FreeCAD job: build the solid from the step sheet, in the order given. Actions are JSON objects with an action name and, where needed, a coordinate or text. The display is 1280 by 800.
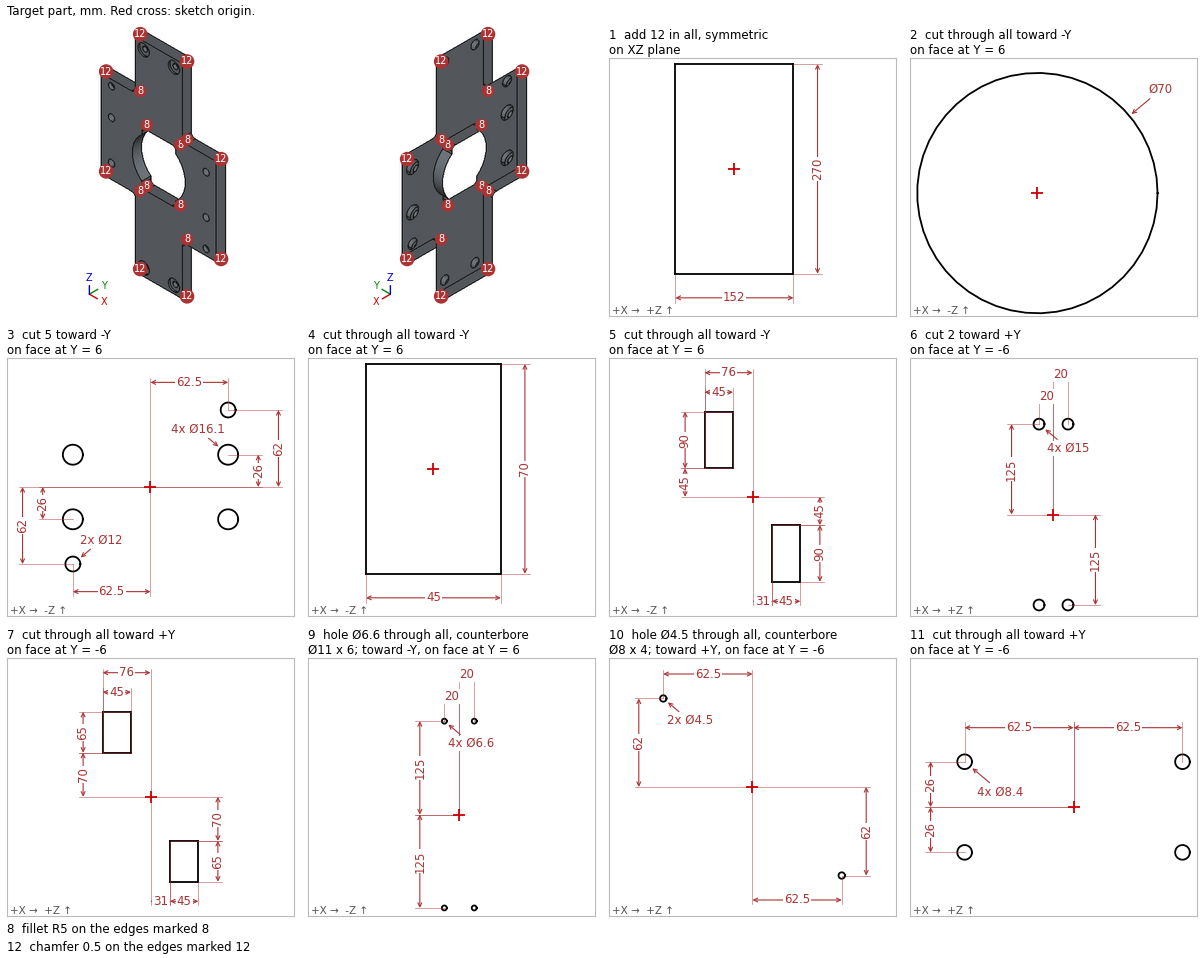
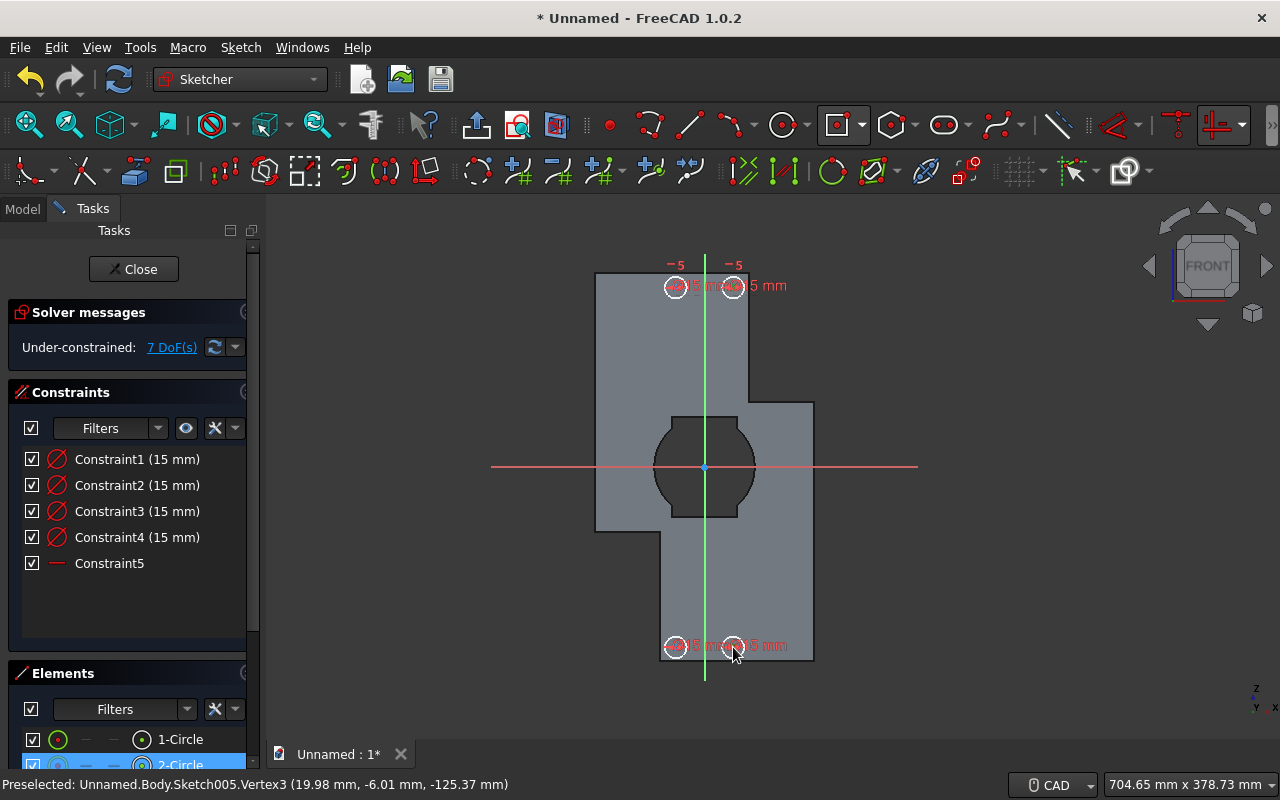
{"action": "key", "text": "v"}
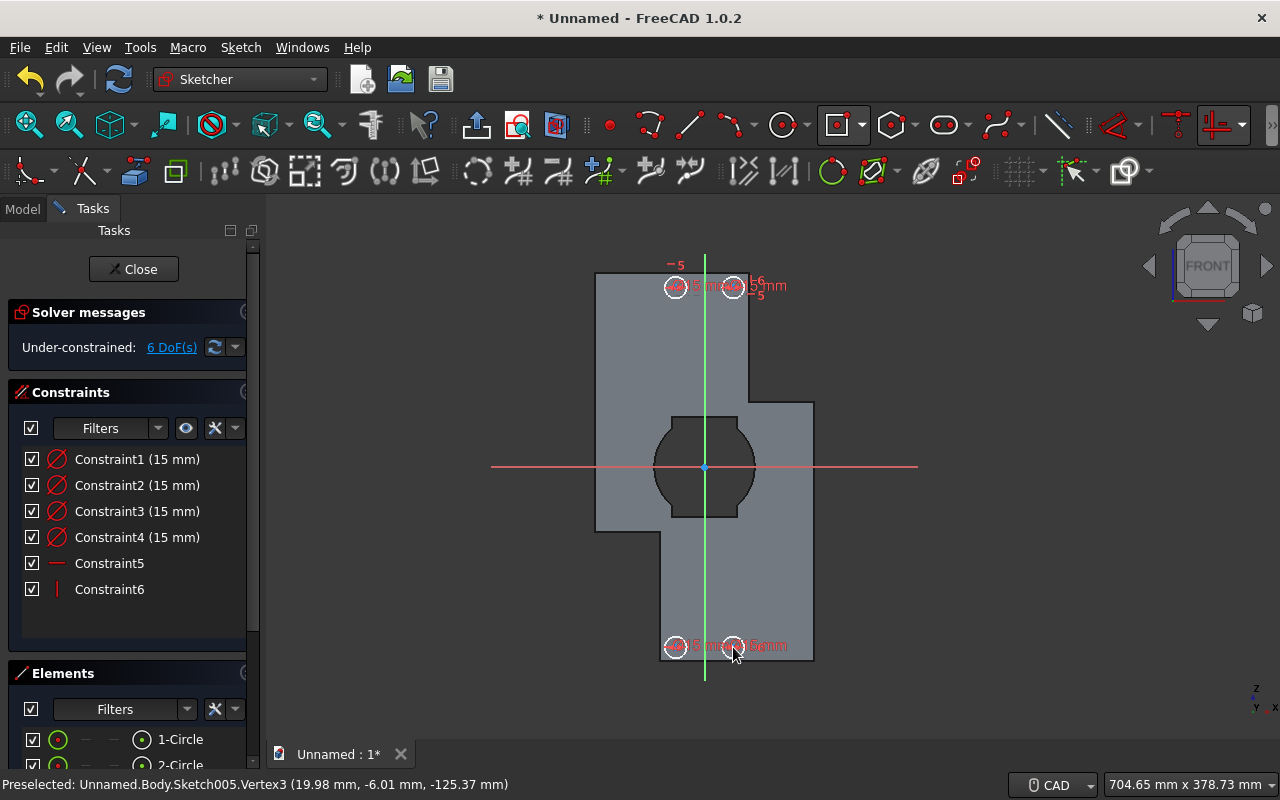
{"action": "left_click", "coordinate": [676, 288]}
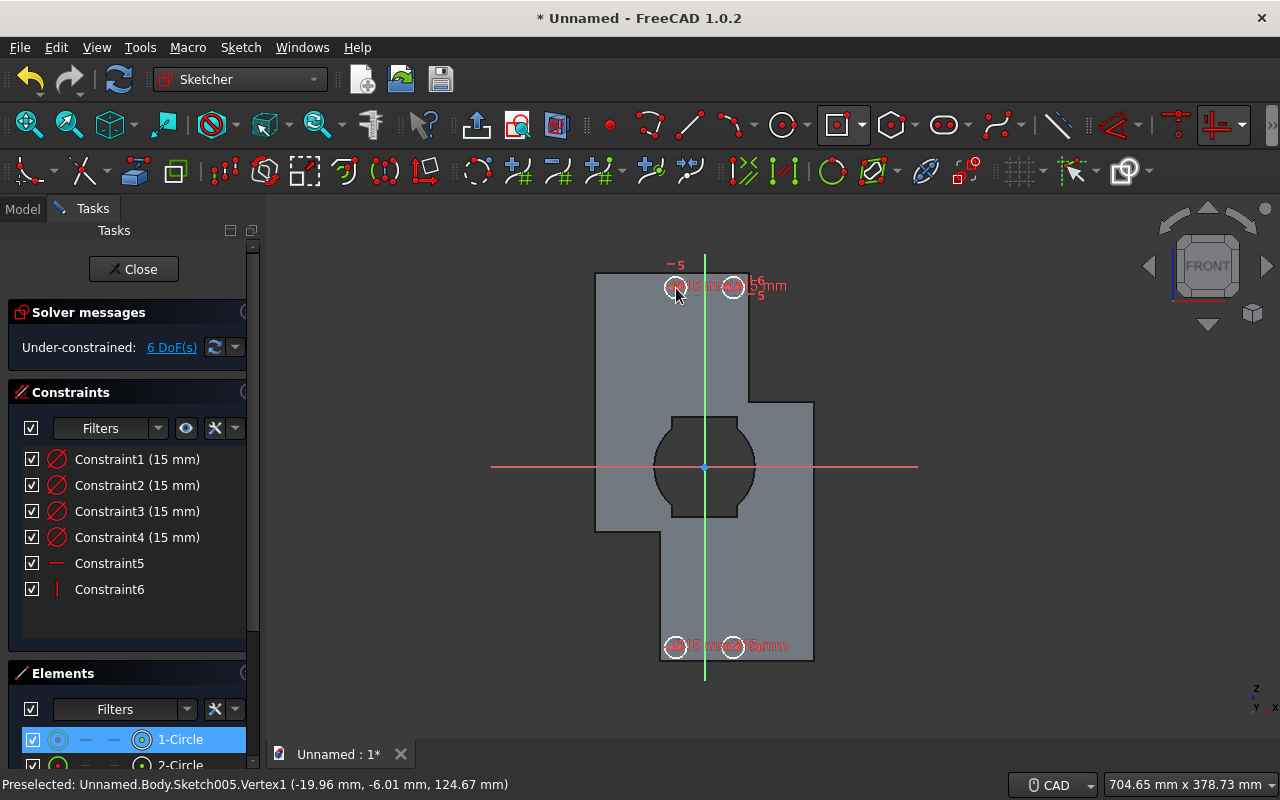
{"action": "left_click", "coordinate": [676, 647]}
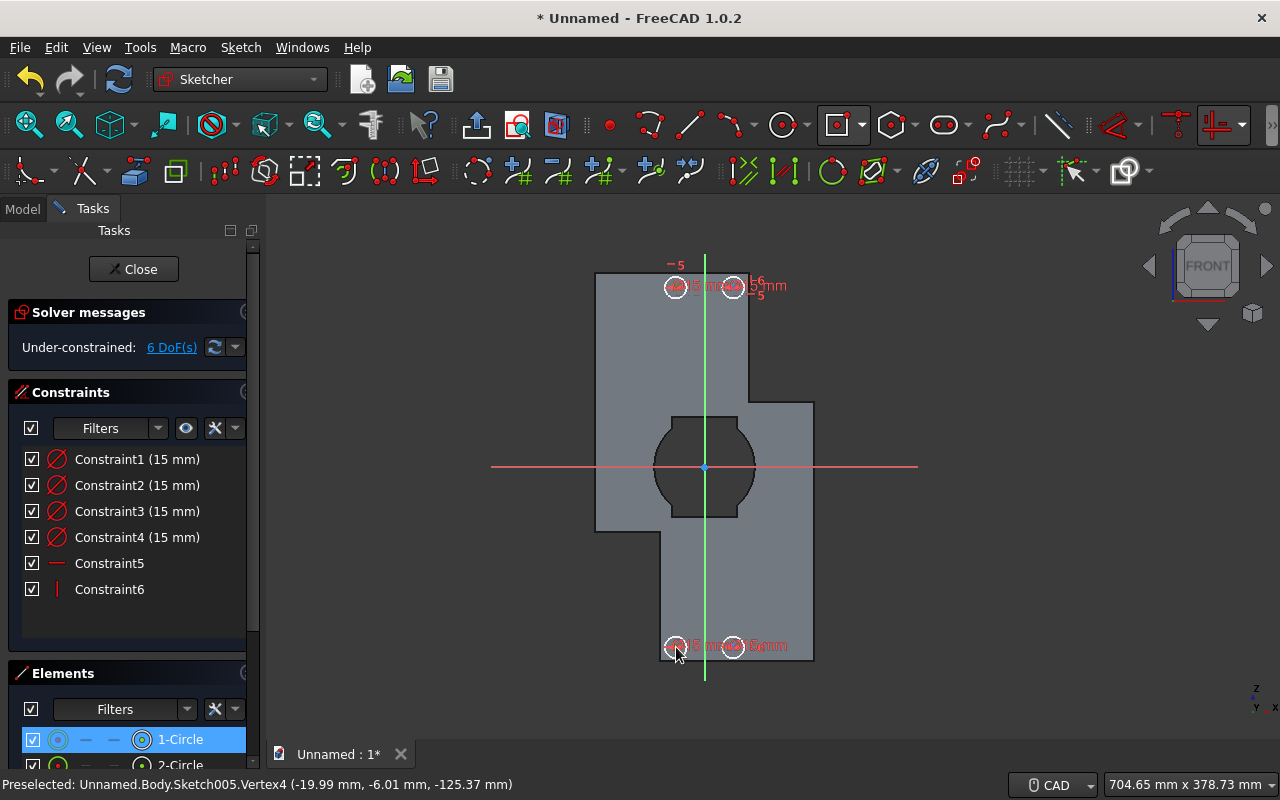
{"action": "key", "text": "v"}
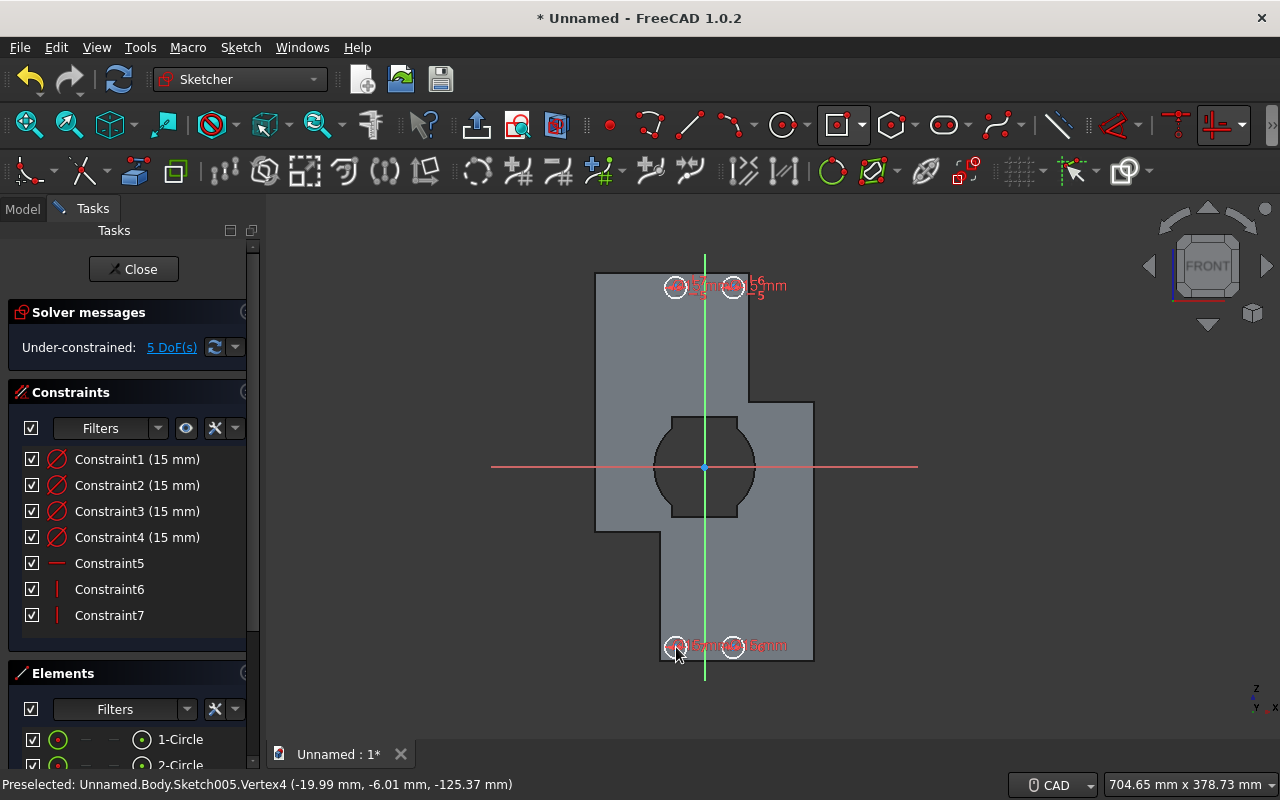
{"action": "left_click", "coordinate": [733, 647]}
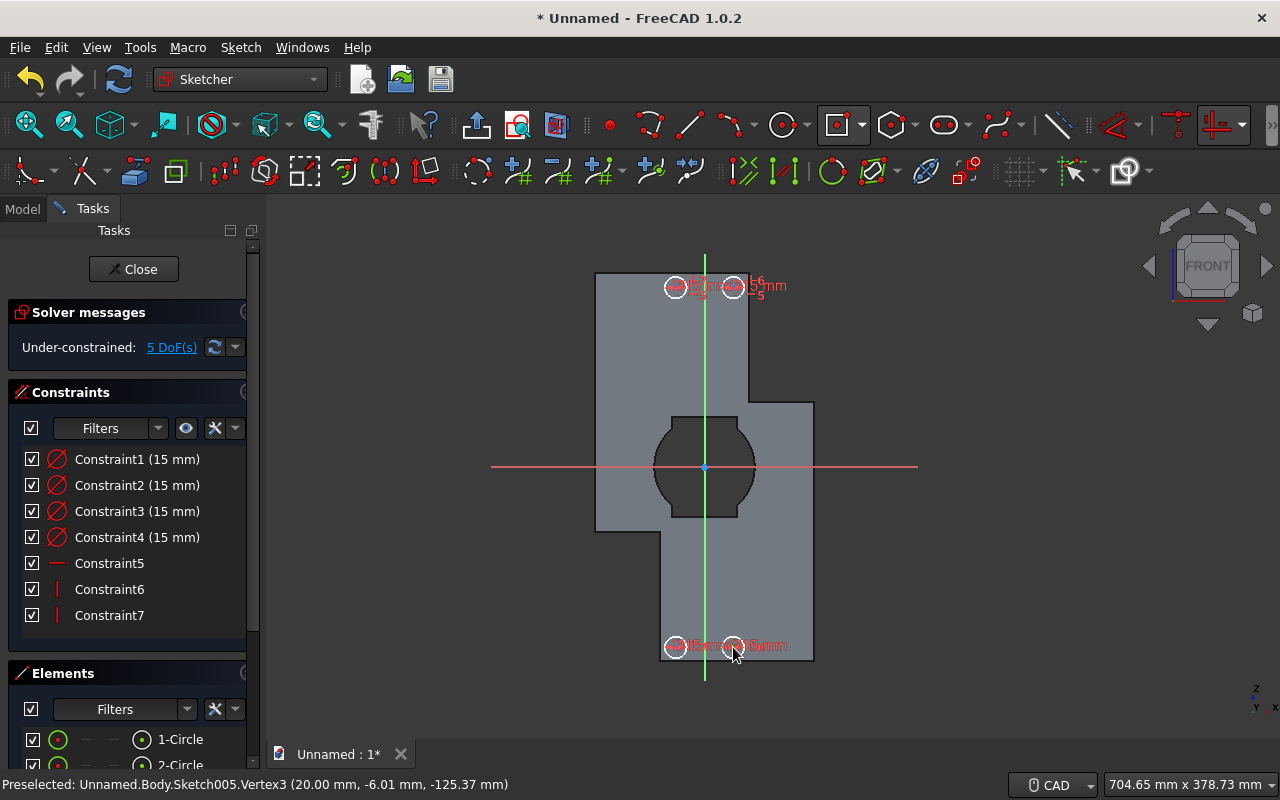
{"action": "left_click", "coordinate": [676, 647]}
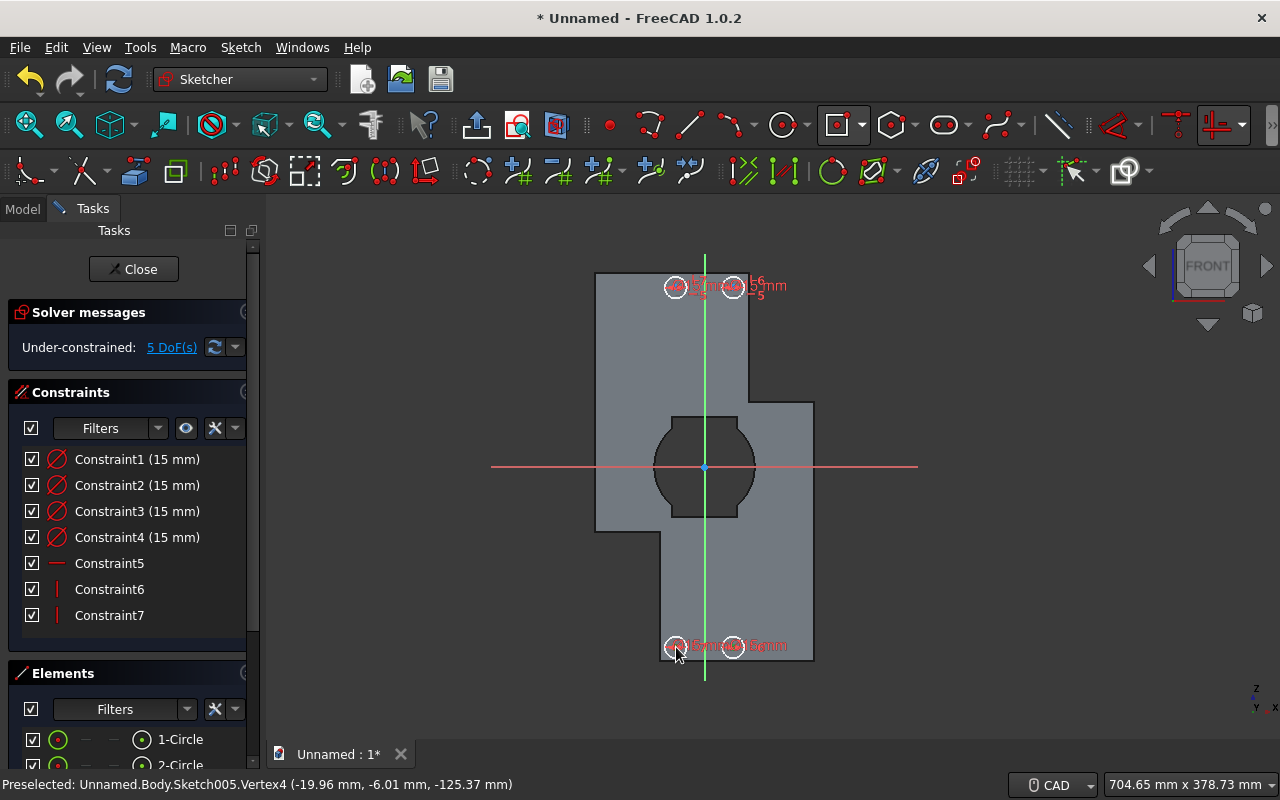
{"action": "key", "text": "h"}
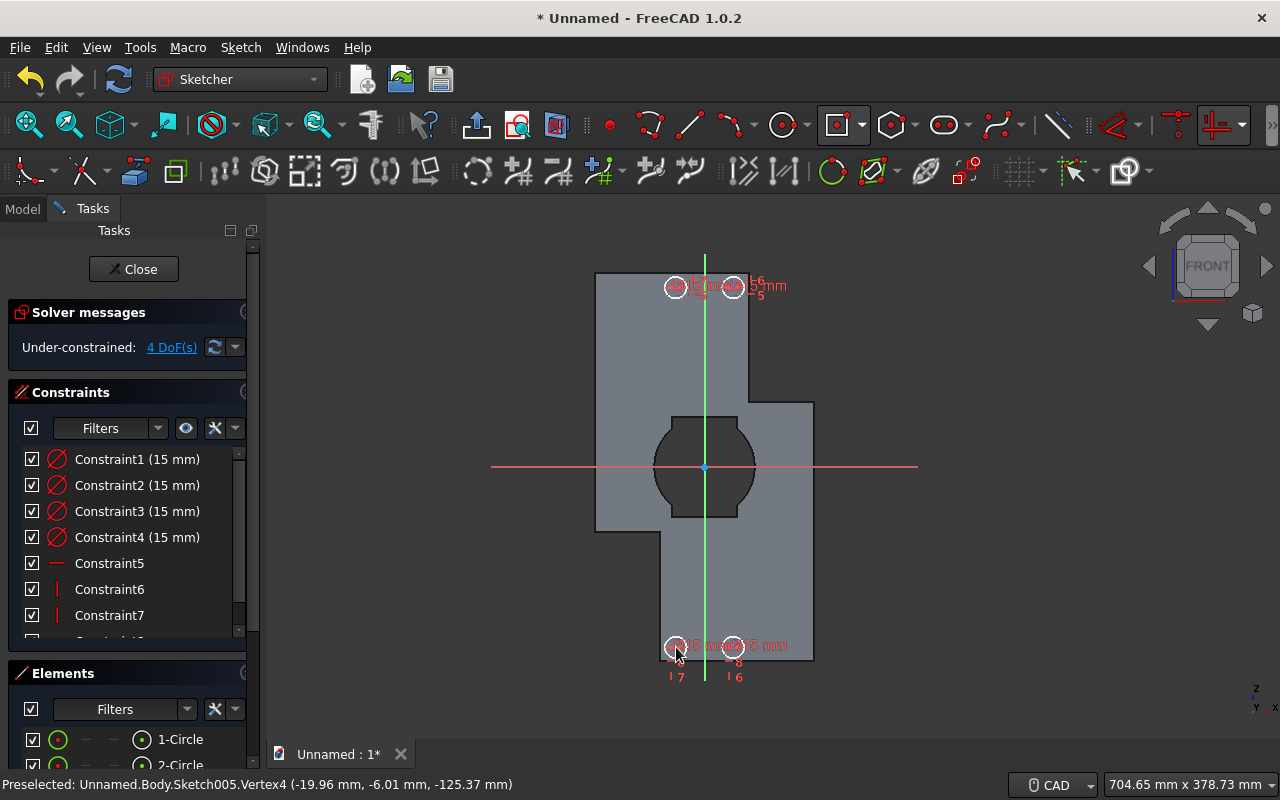
{"action": "key", "text": "d"}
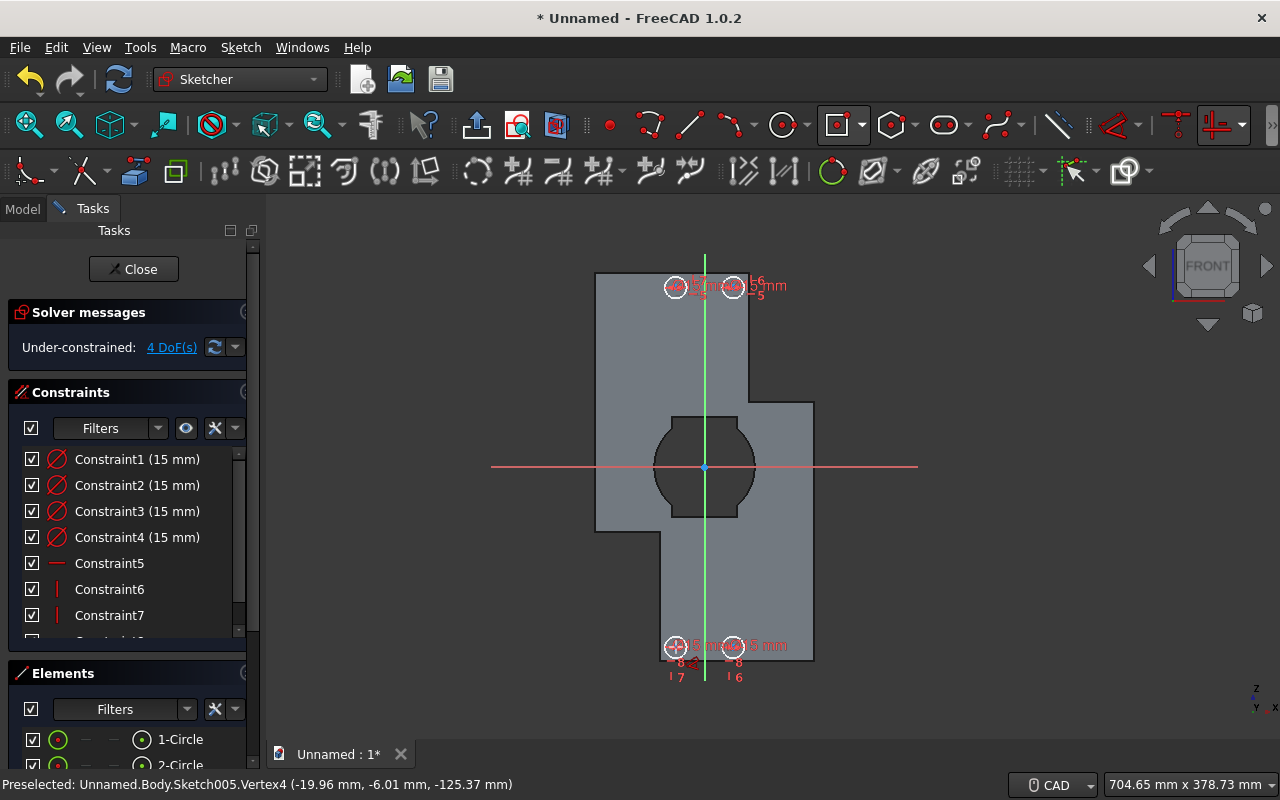
{"action": "scroll", "coordinate": [676, 288], "scroll_direction": "up", "scroll_amount": 2}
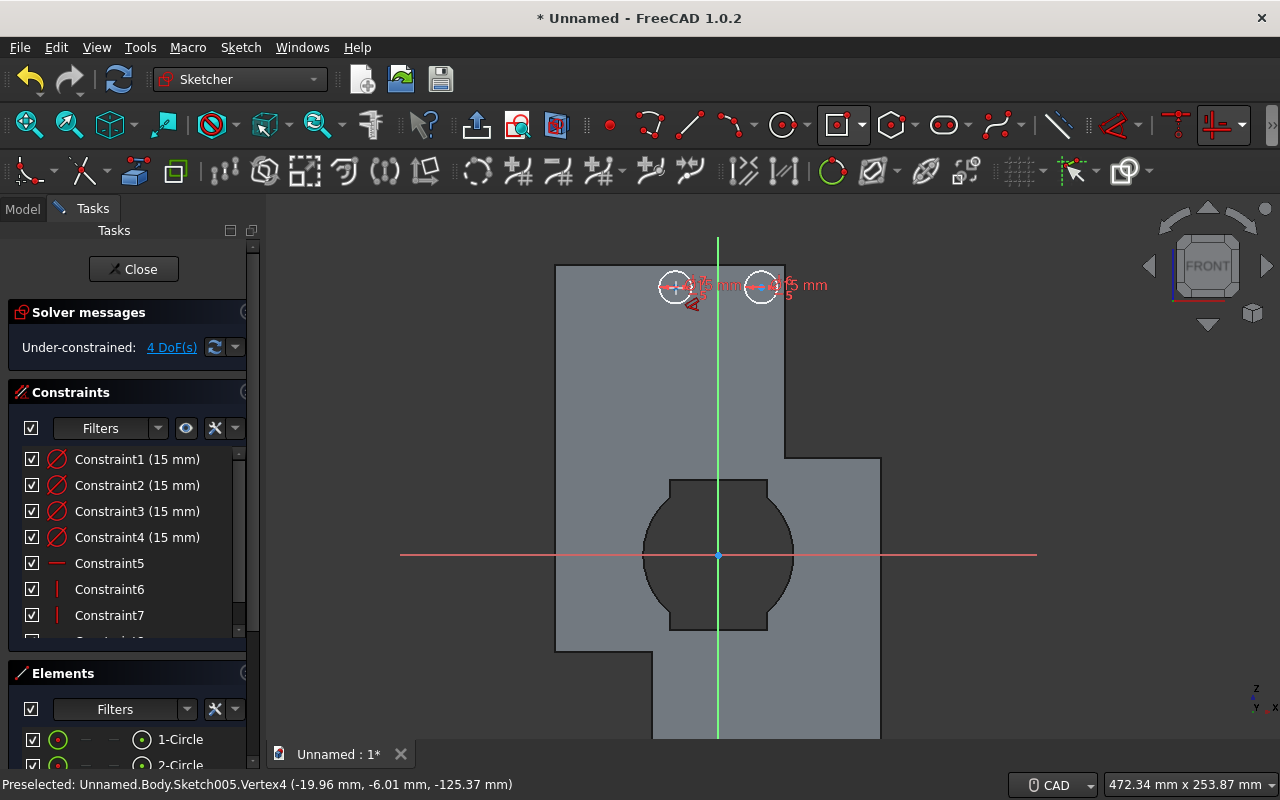
{"action": "left_click", "coordinate": [675, 287]}
{"action": "left_click", "coordinate": [697, 253]}